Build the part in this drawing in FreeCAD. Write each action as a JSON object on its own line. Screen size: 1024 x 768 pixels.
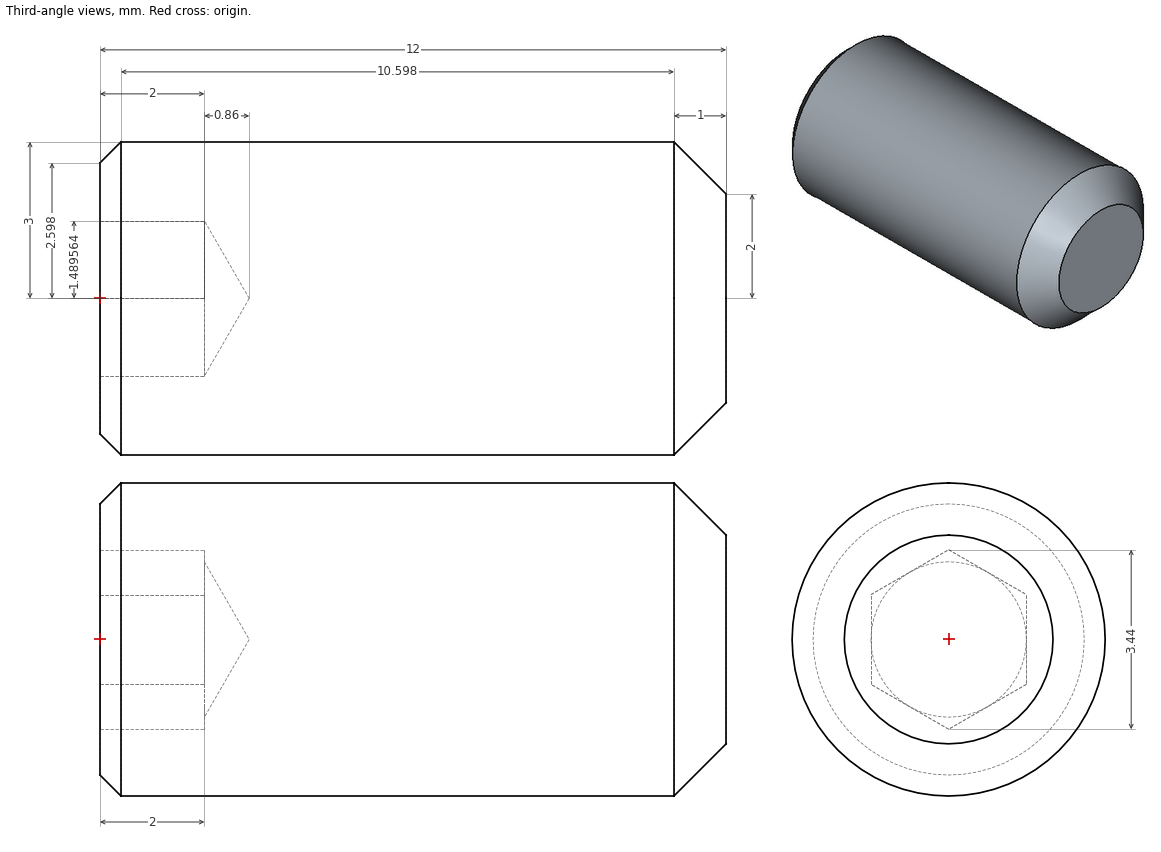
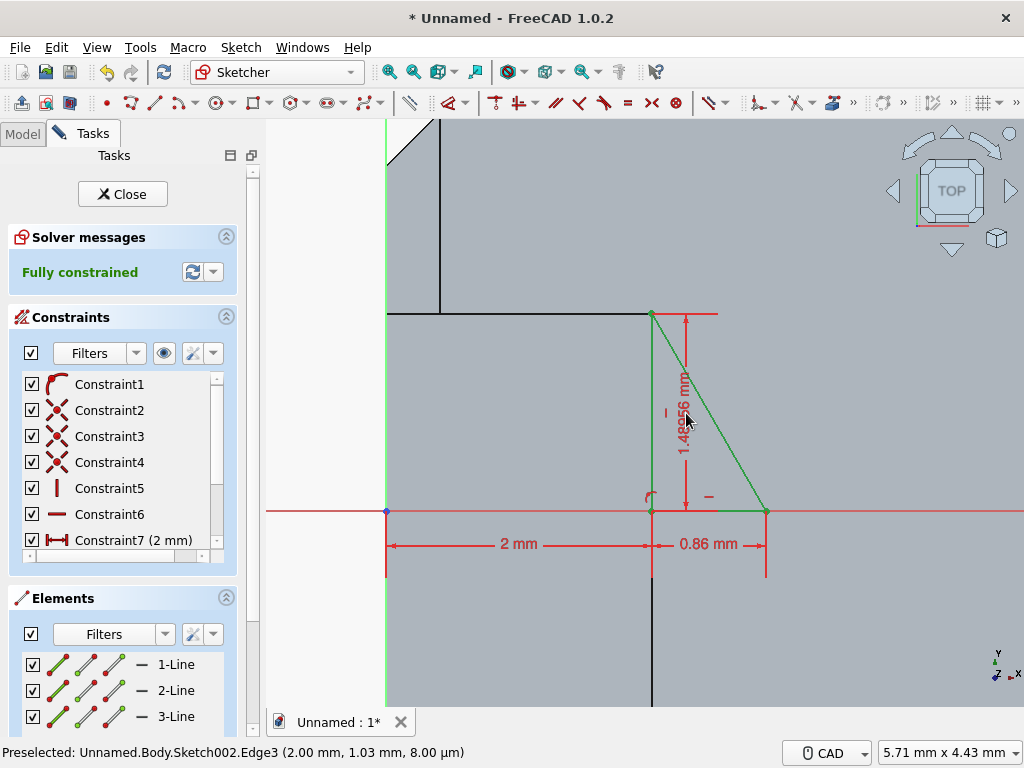
{"action": "left_click", "coordinate": [123, 194]}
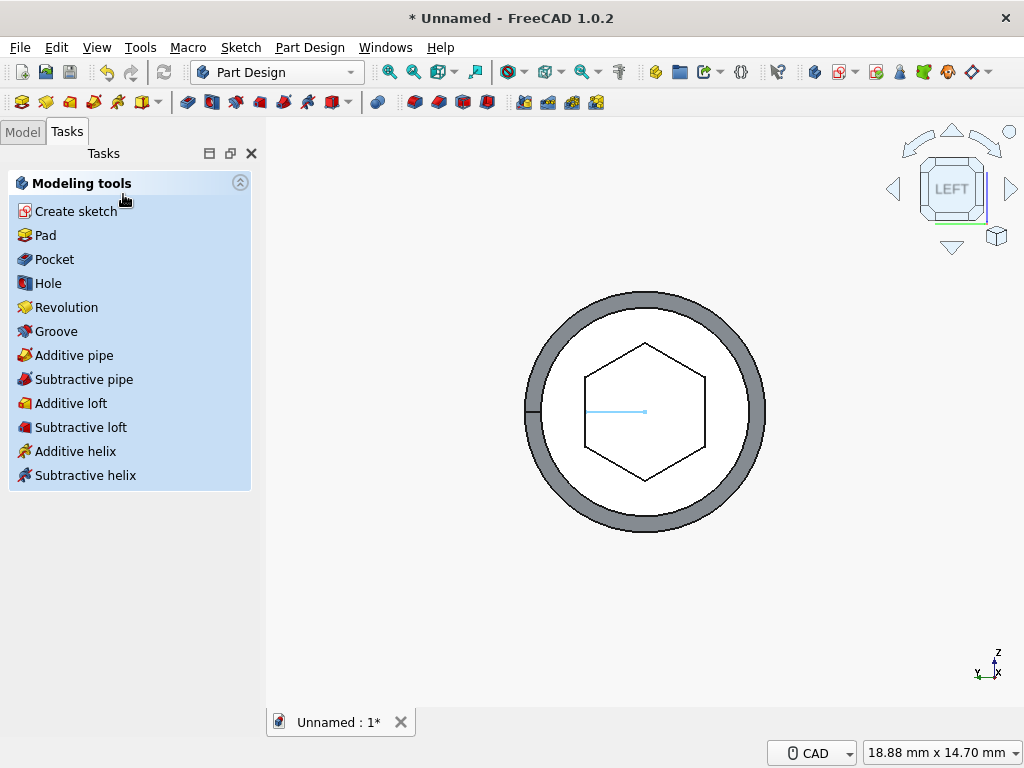
{"action": "left_click", "coordinate": [236, 102]}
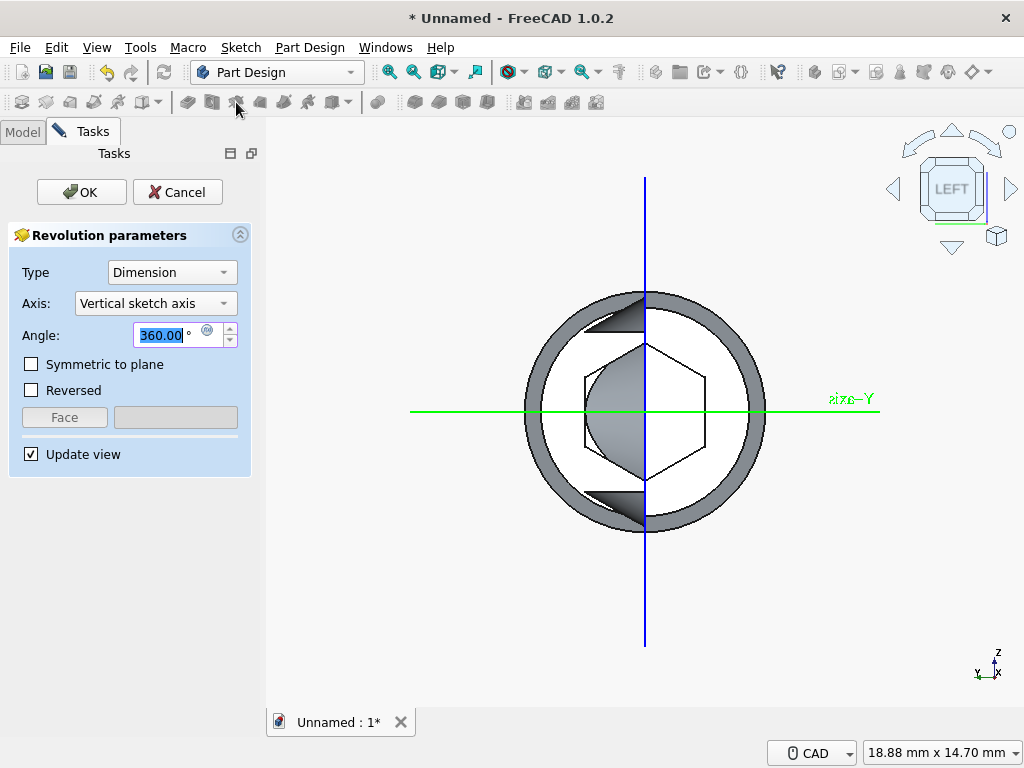
{"action": "left_click", "coordinate": [156, 304]}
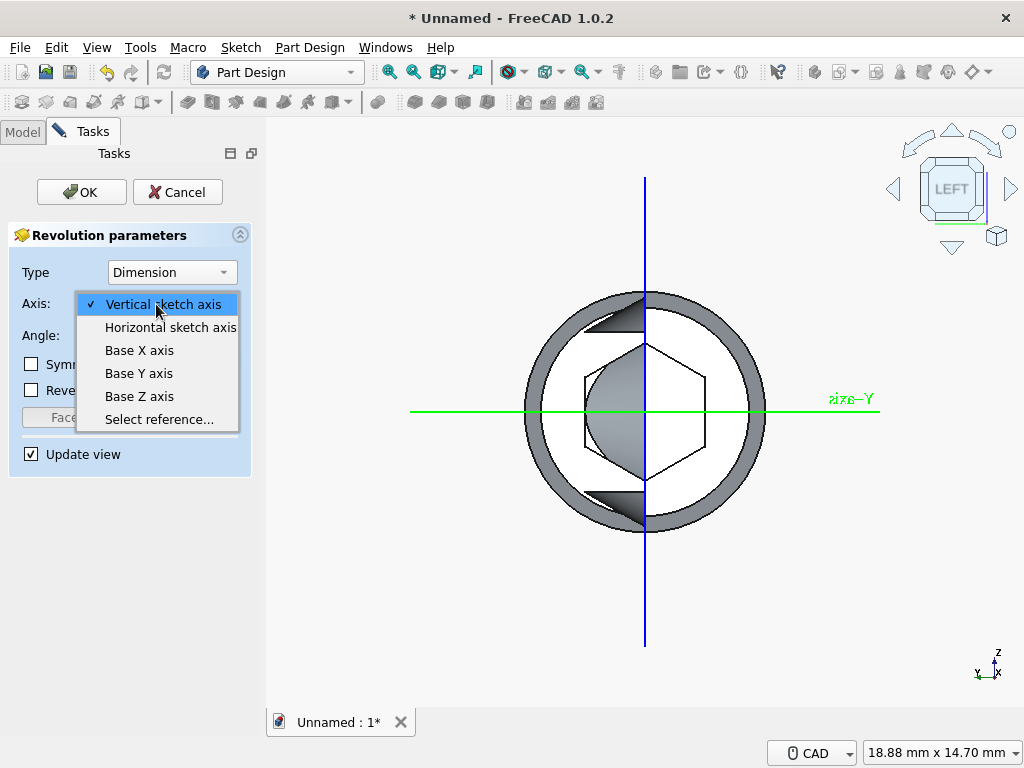
{"action": "left_click", "coordinate": [156, 328]}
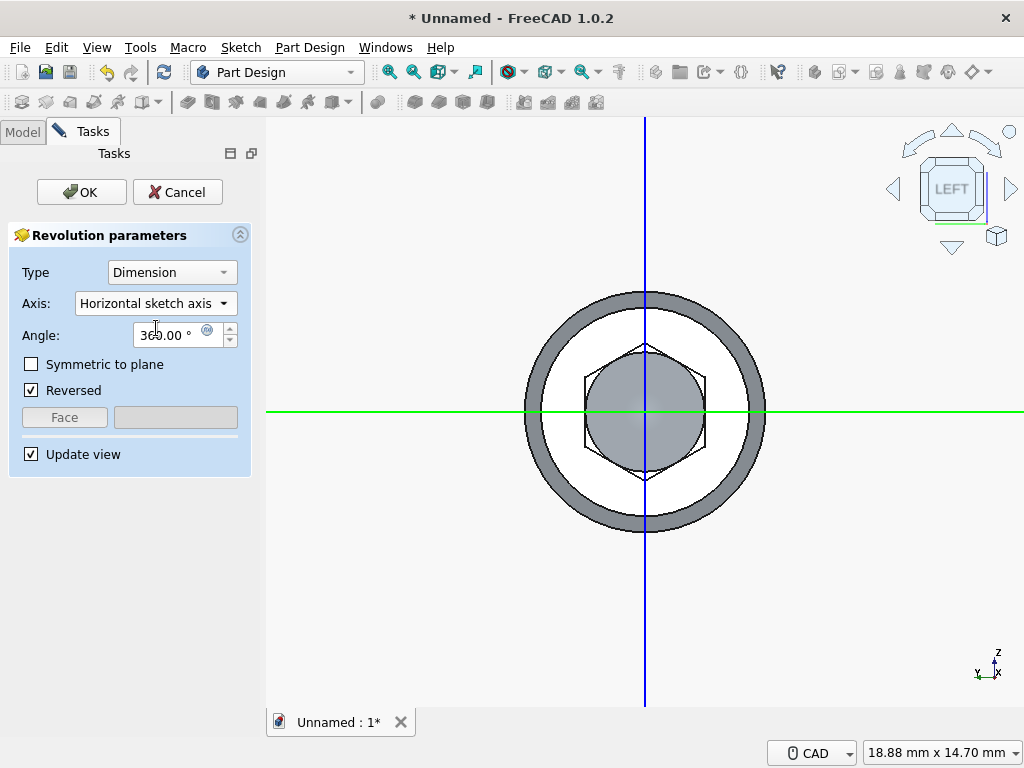
{"action": "left_click", "coordinate": [82, 192]}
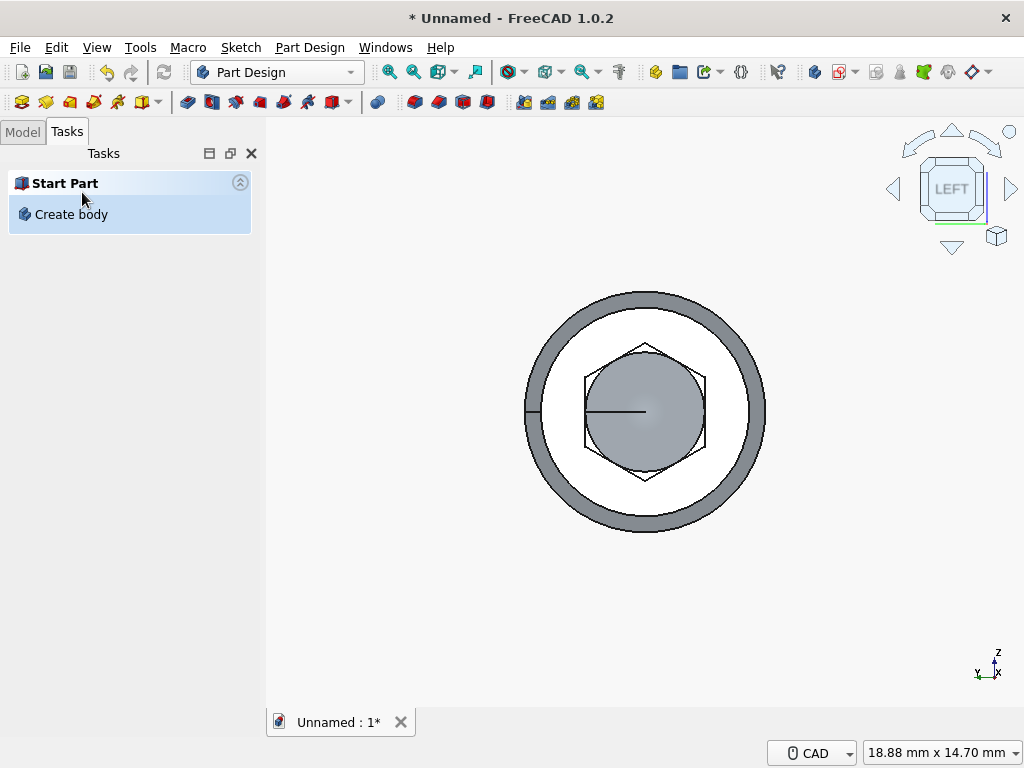
{"action": "key", "text": "0"}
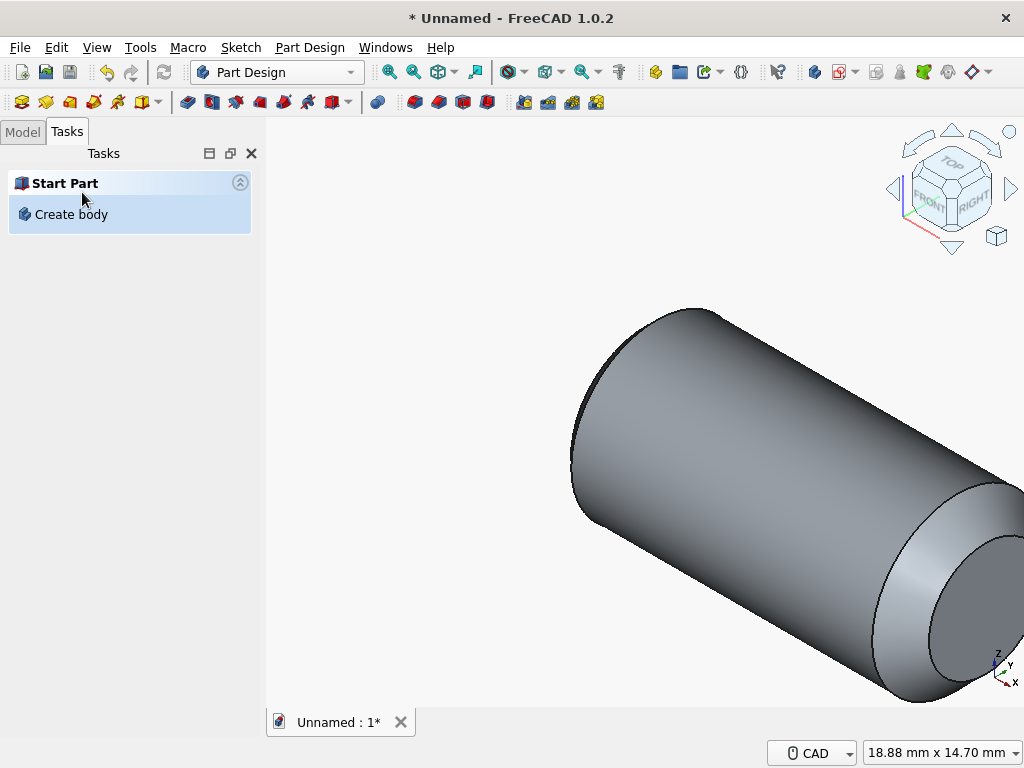
{"action": "key", "text": "v f"}